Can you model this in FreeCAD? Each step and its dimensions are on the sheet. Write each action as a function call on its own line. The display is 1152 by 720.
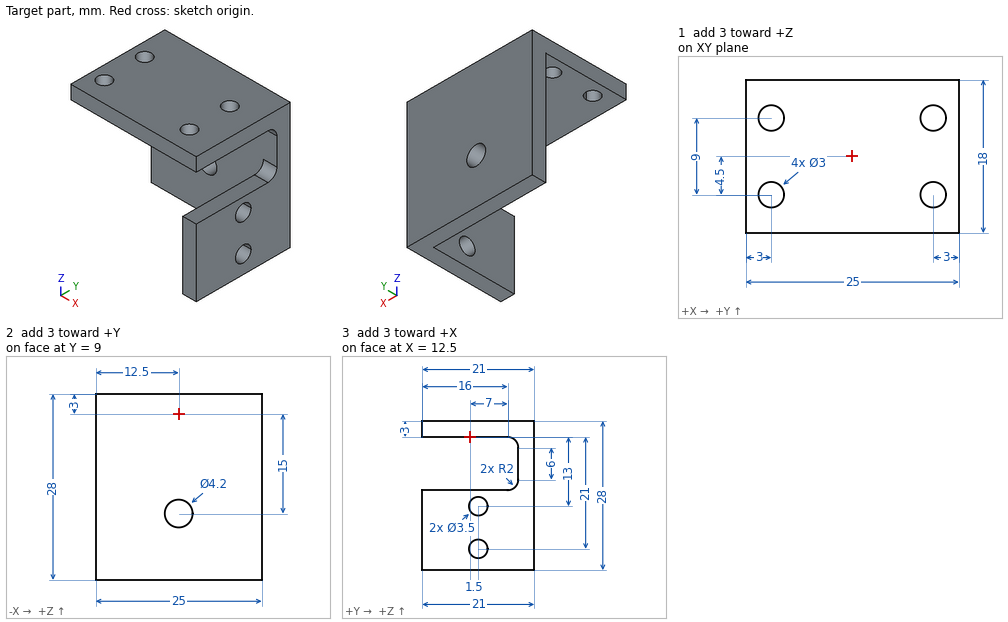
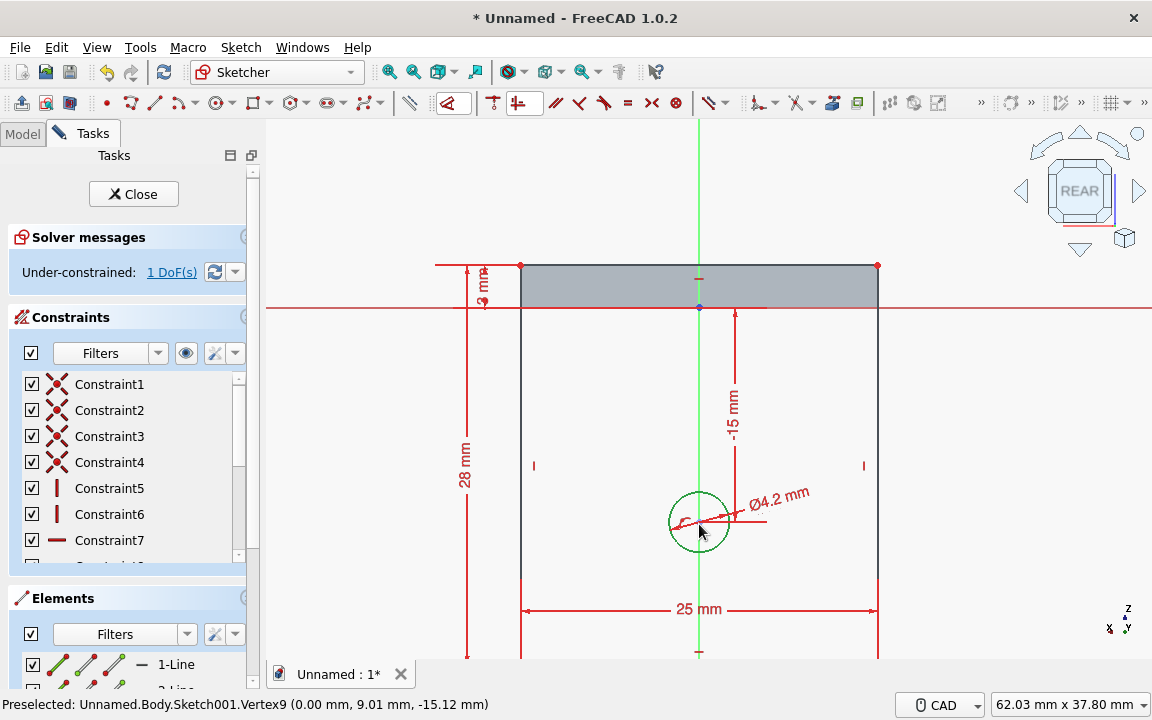
click(521, 265)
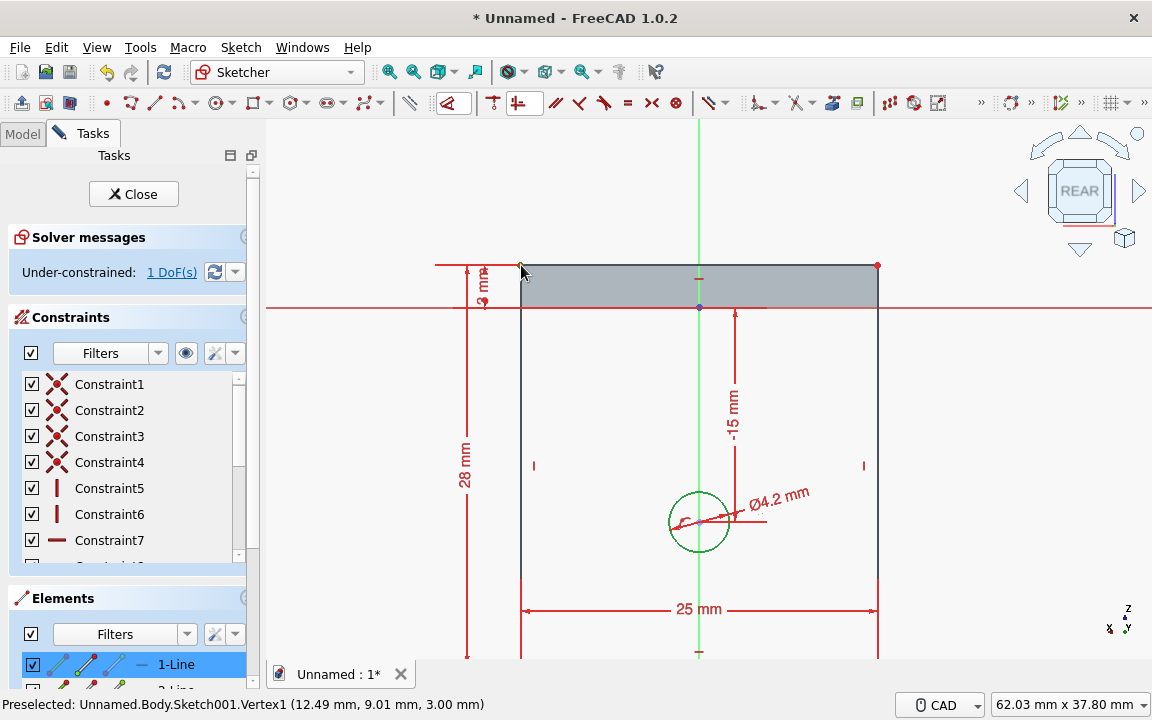
key(l)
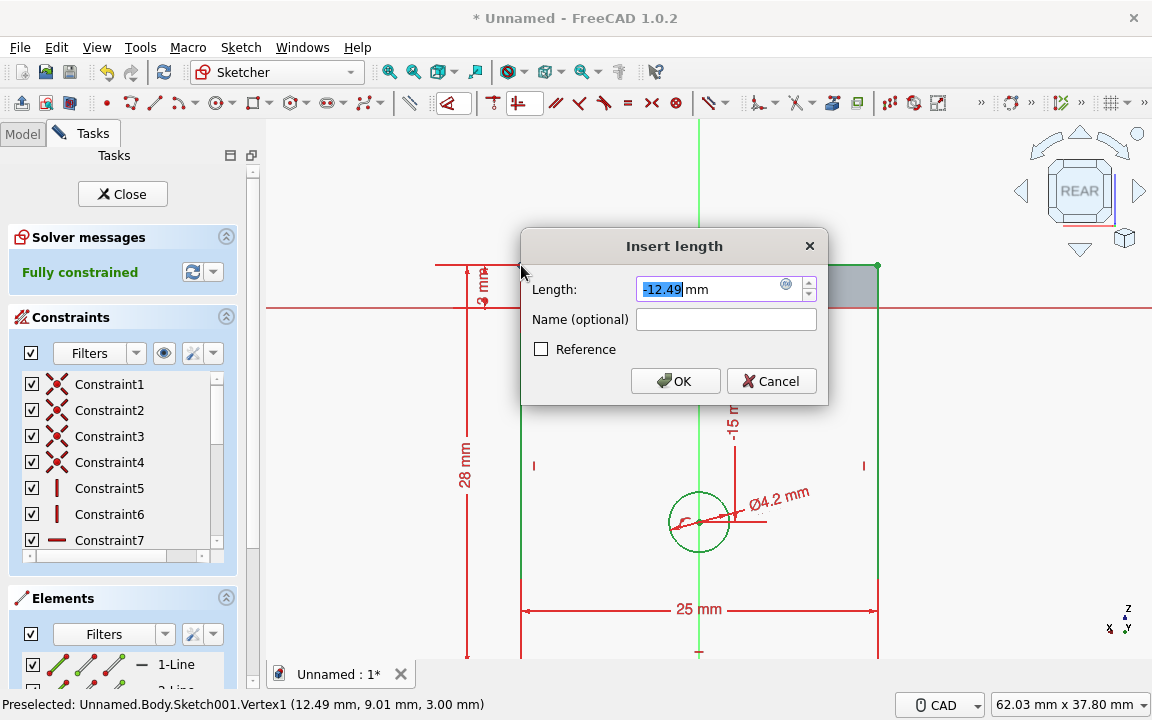
text(-12.5)
key(Return)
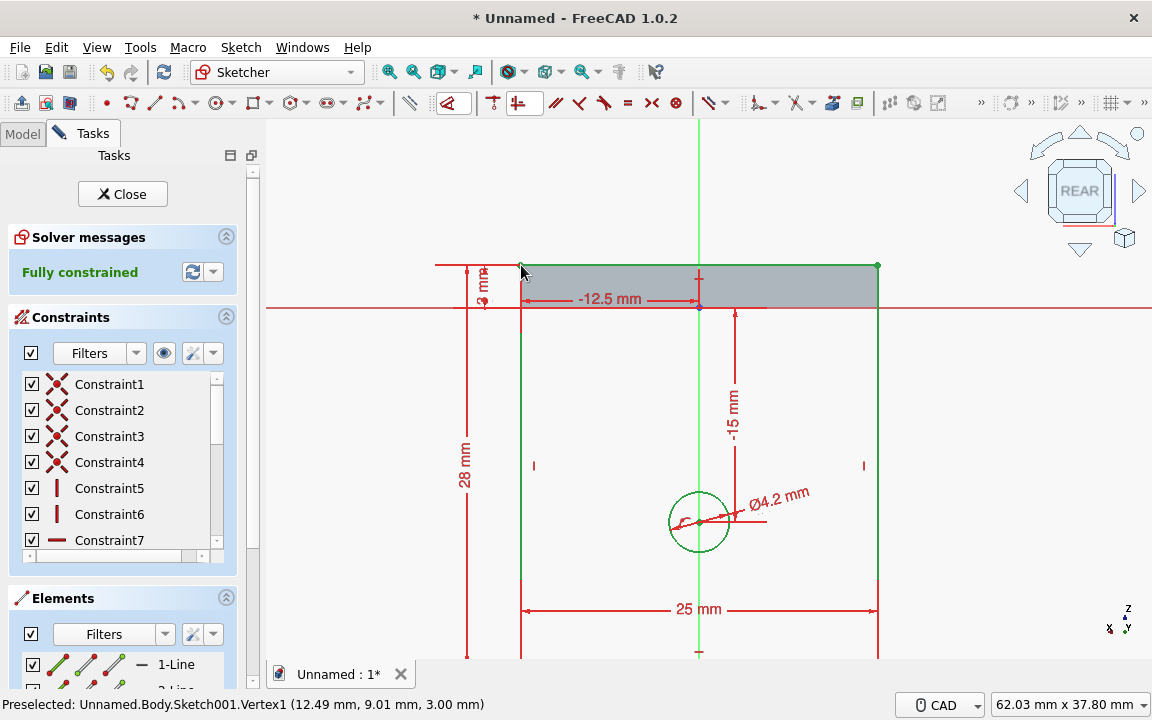
click(123, 194)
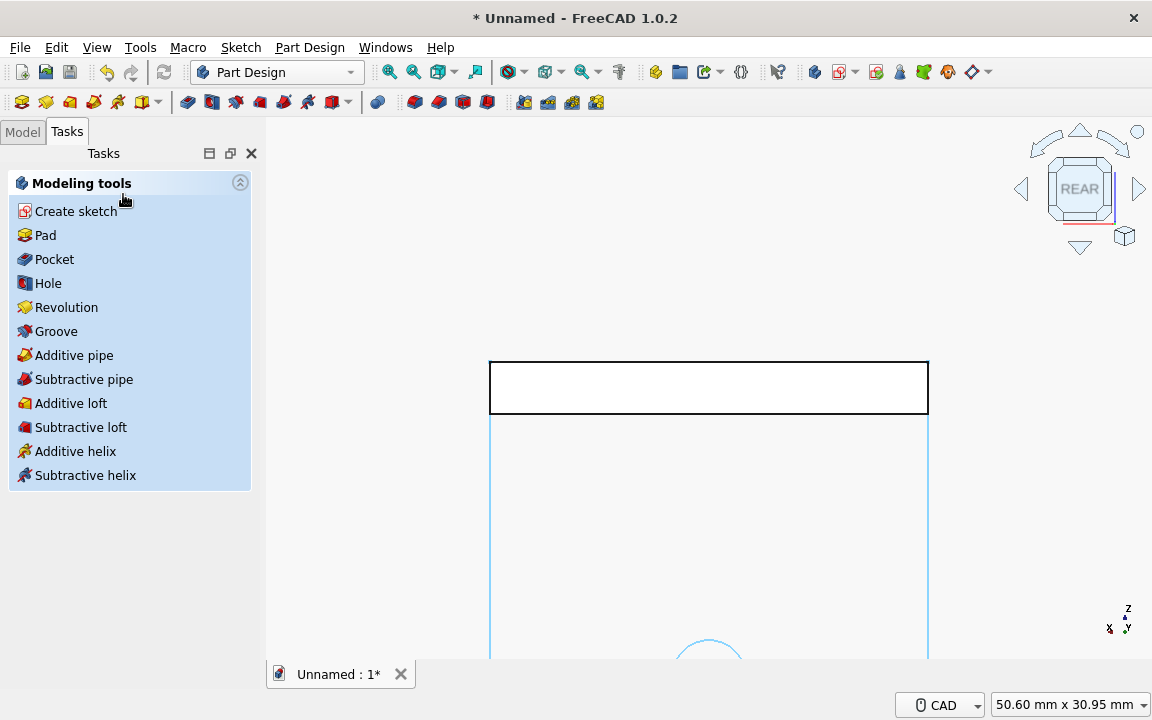
click(22, 102)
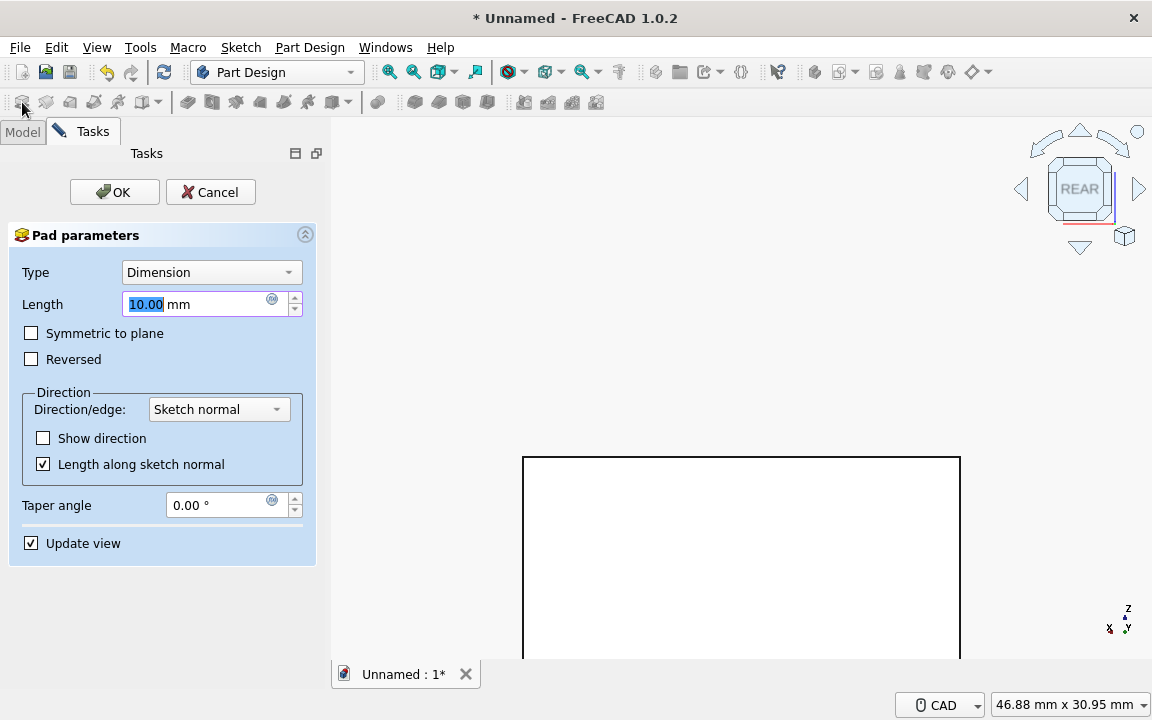
text(3)
key(Tab)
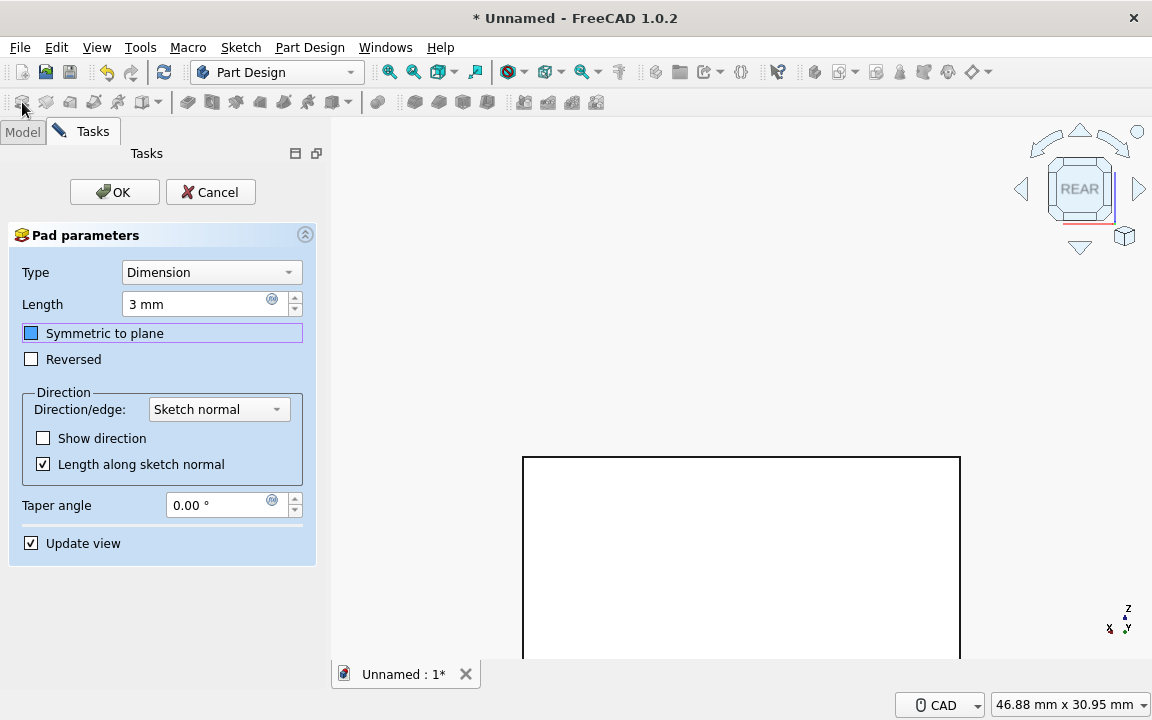
click(115, 192)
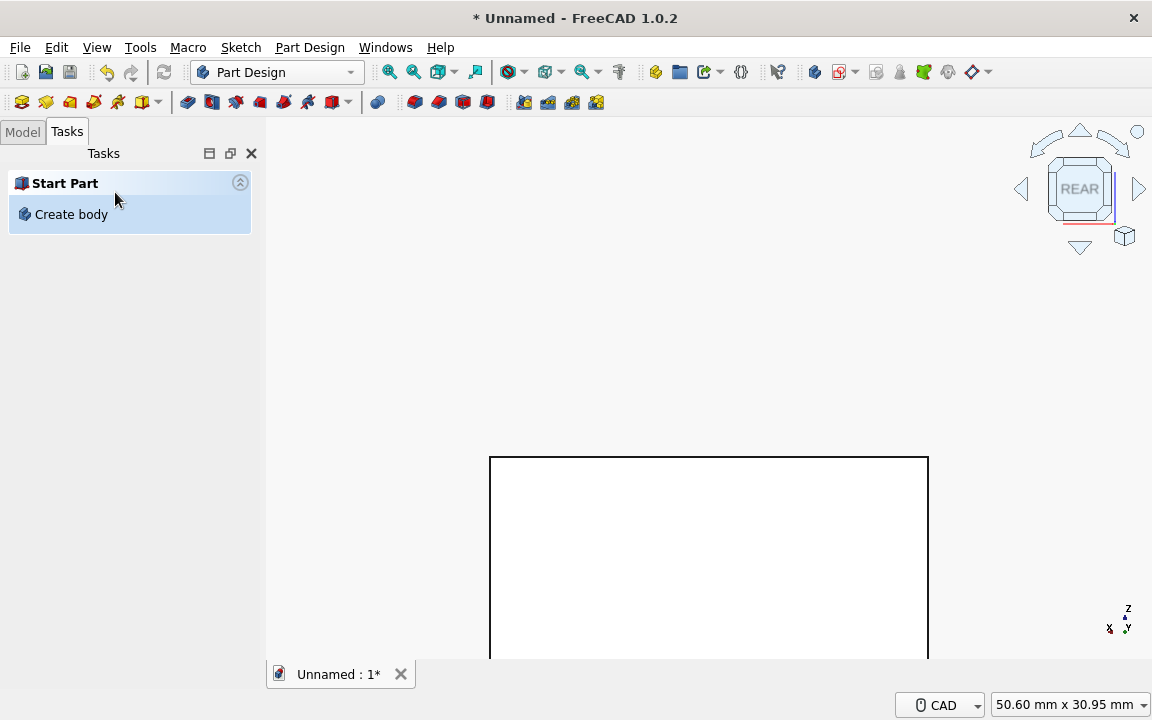
key(v)
key(f)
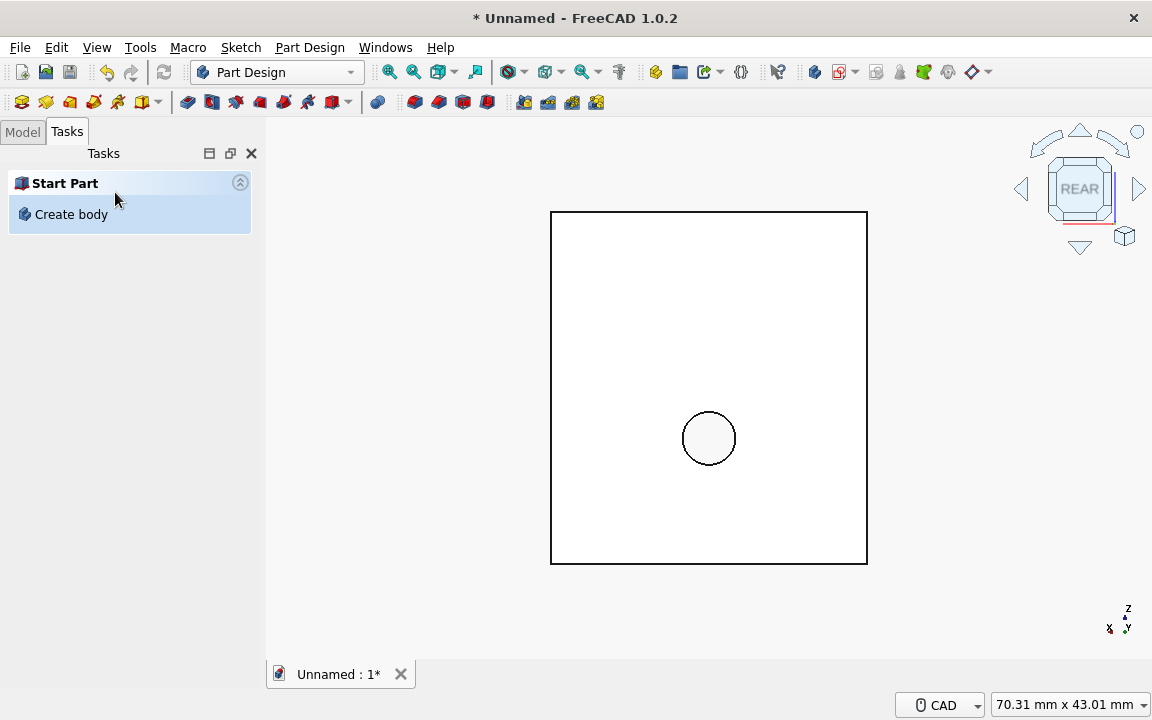
key(0)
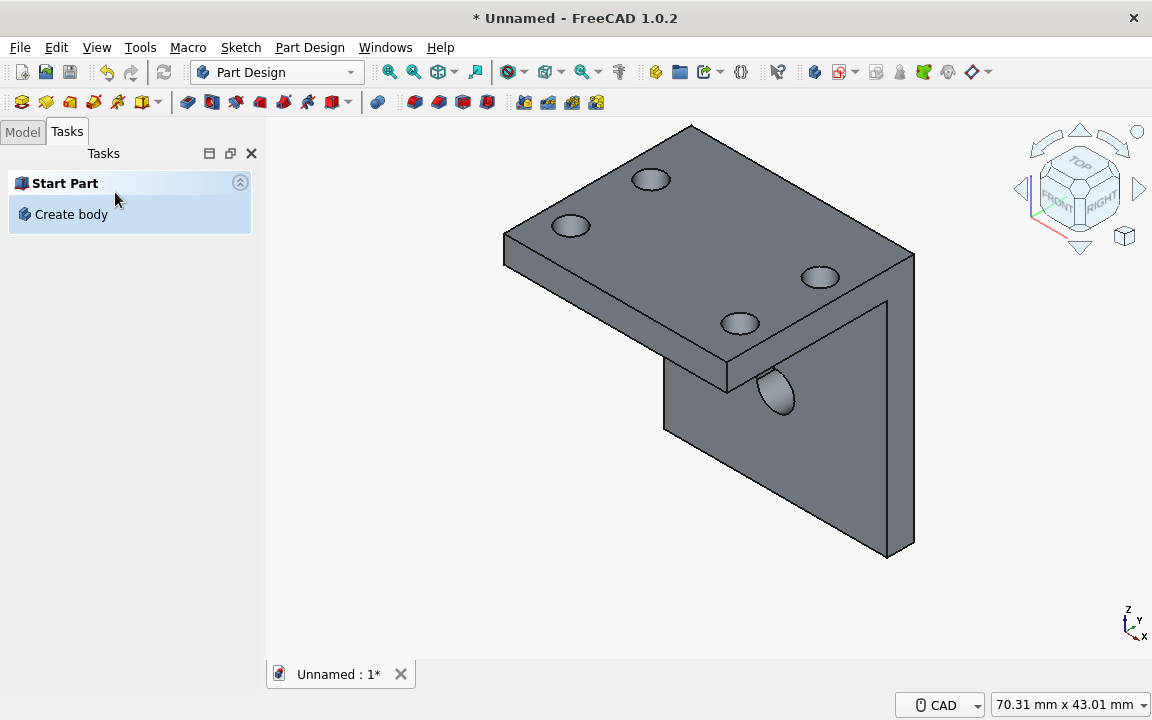
click(901, 282)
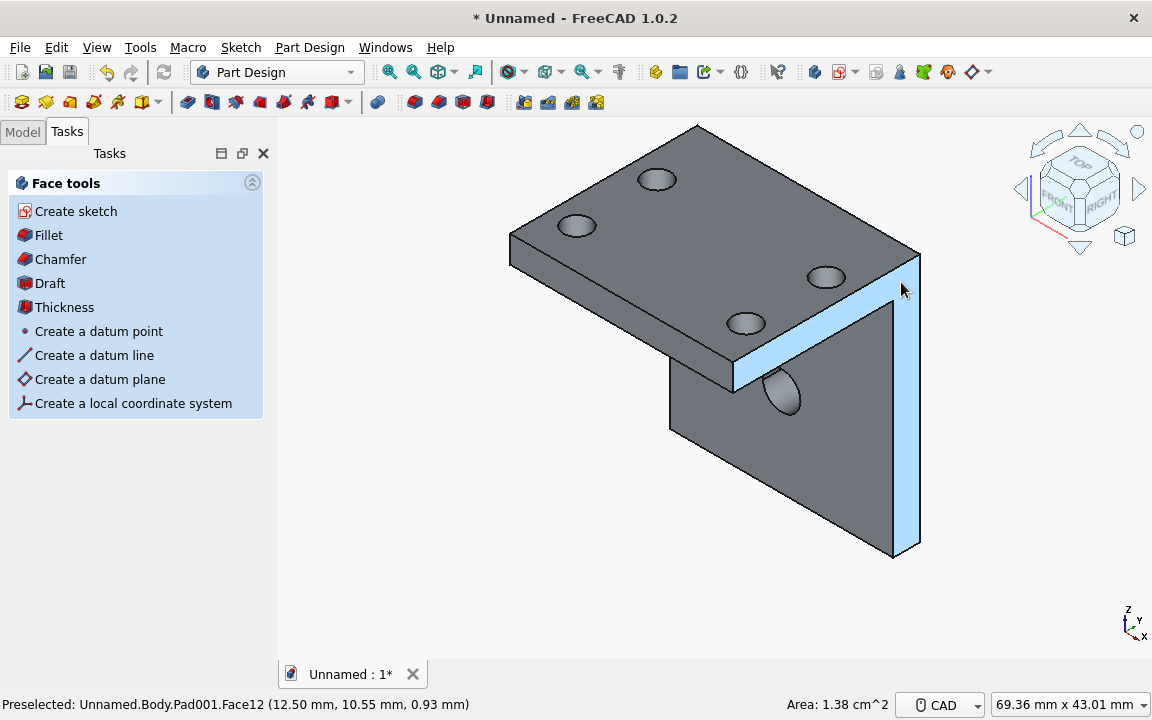
click(840, 72)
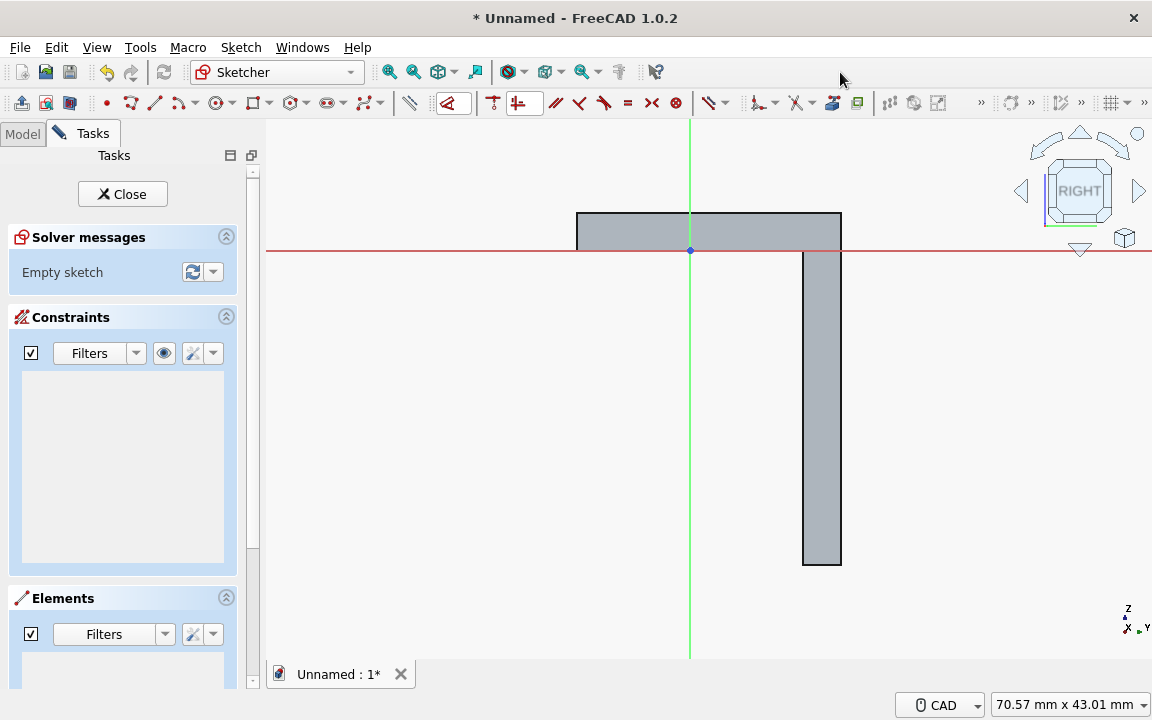
click(132, 104)